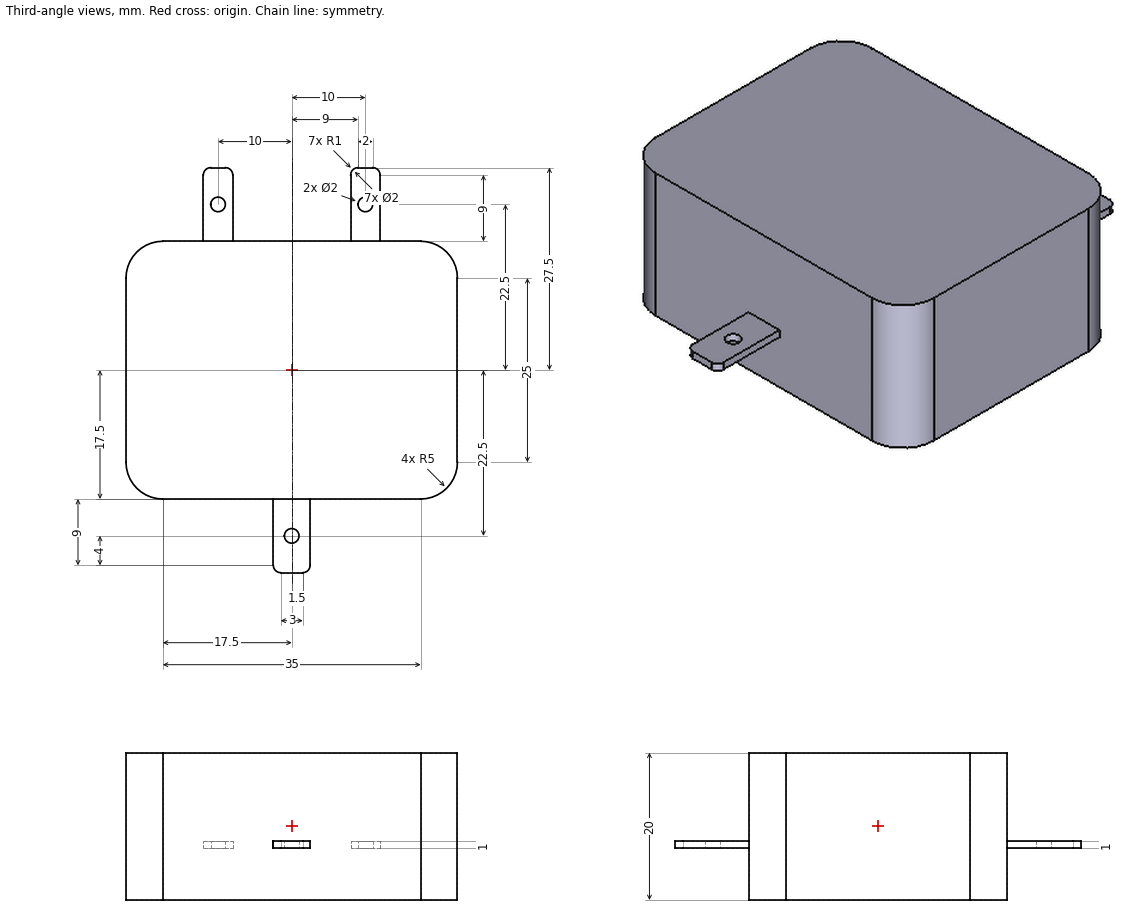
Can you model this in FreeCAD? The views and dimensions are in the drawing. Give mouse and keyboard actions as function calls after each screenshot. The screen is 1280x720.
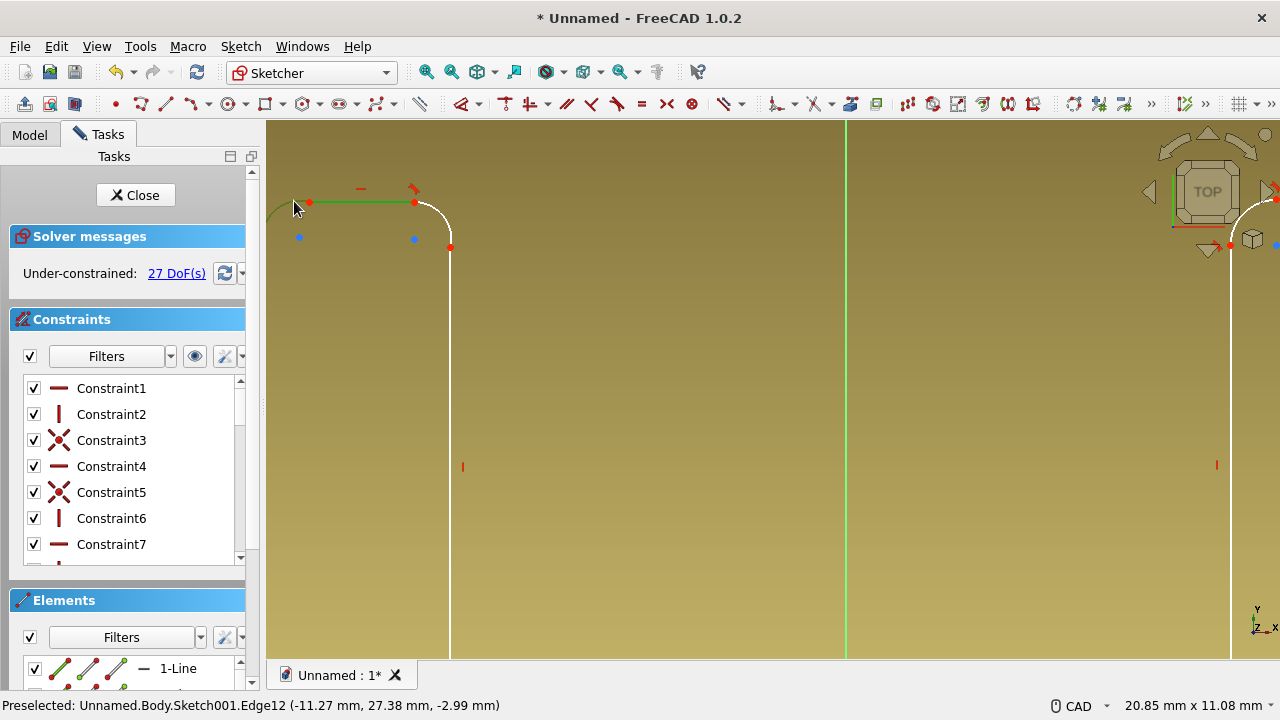
click(617, 104)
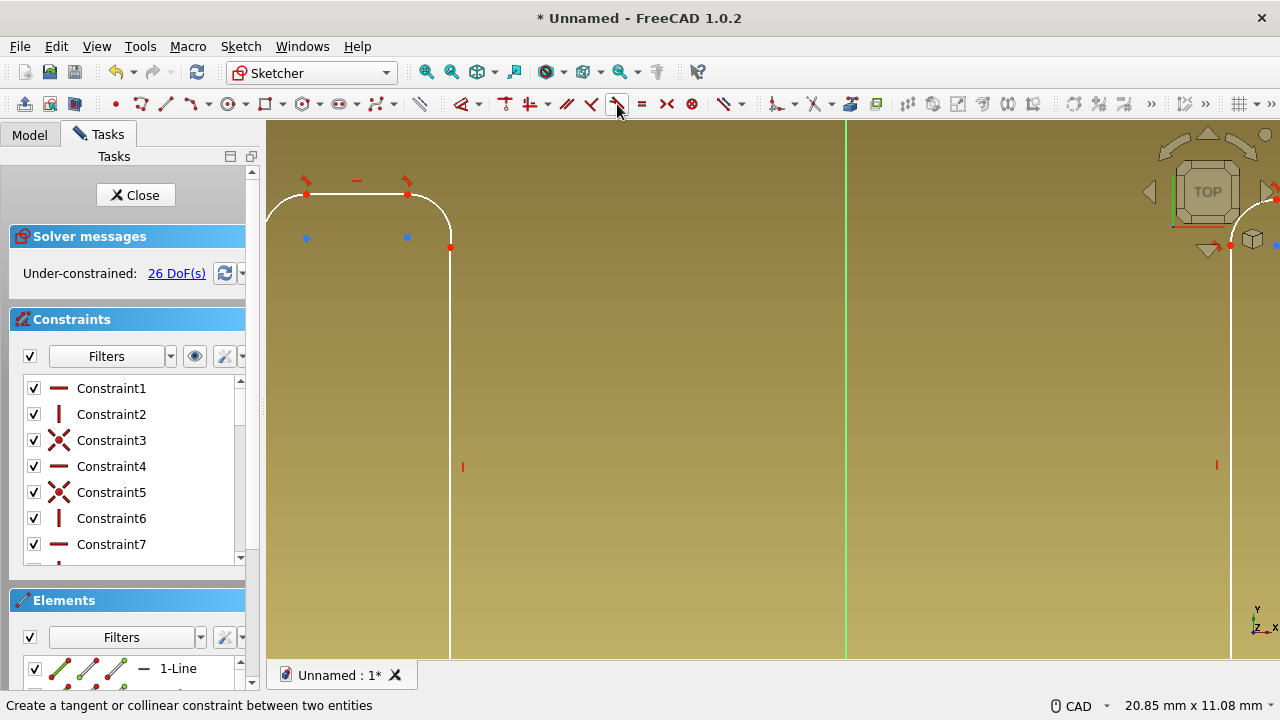
scroll(682, 211, down, 10)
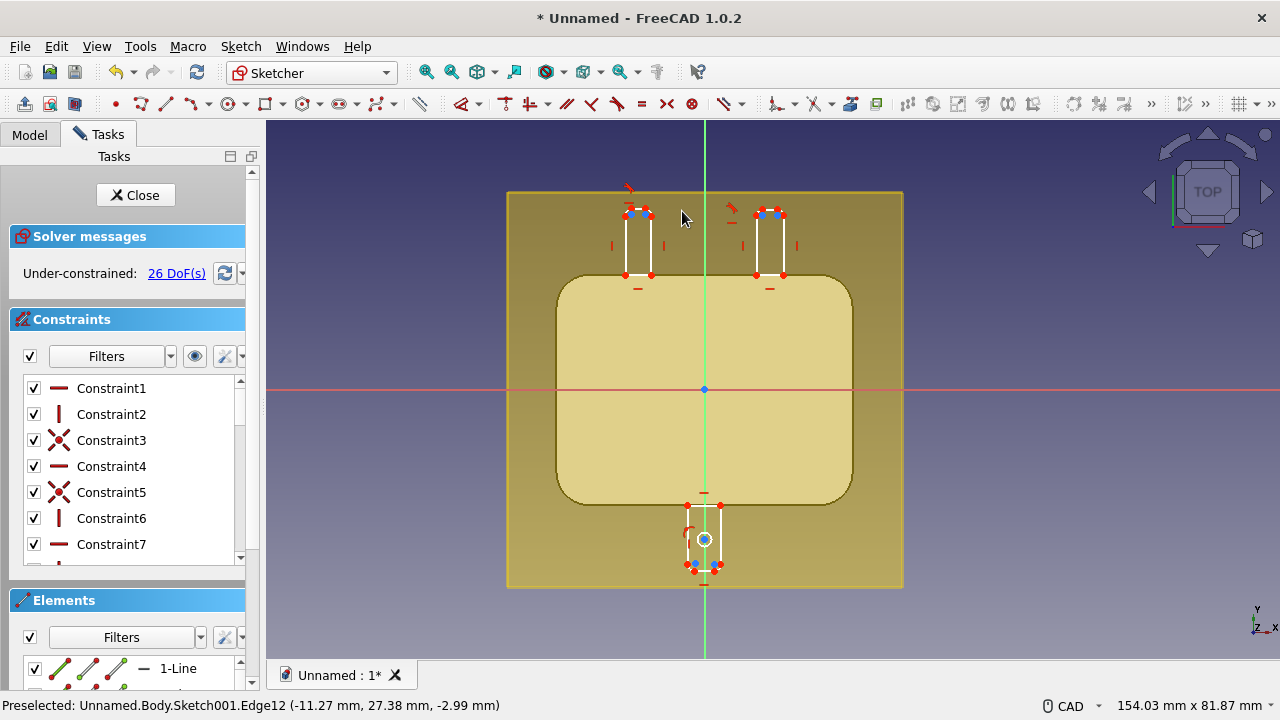
click(651, 234)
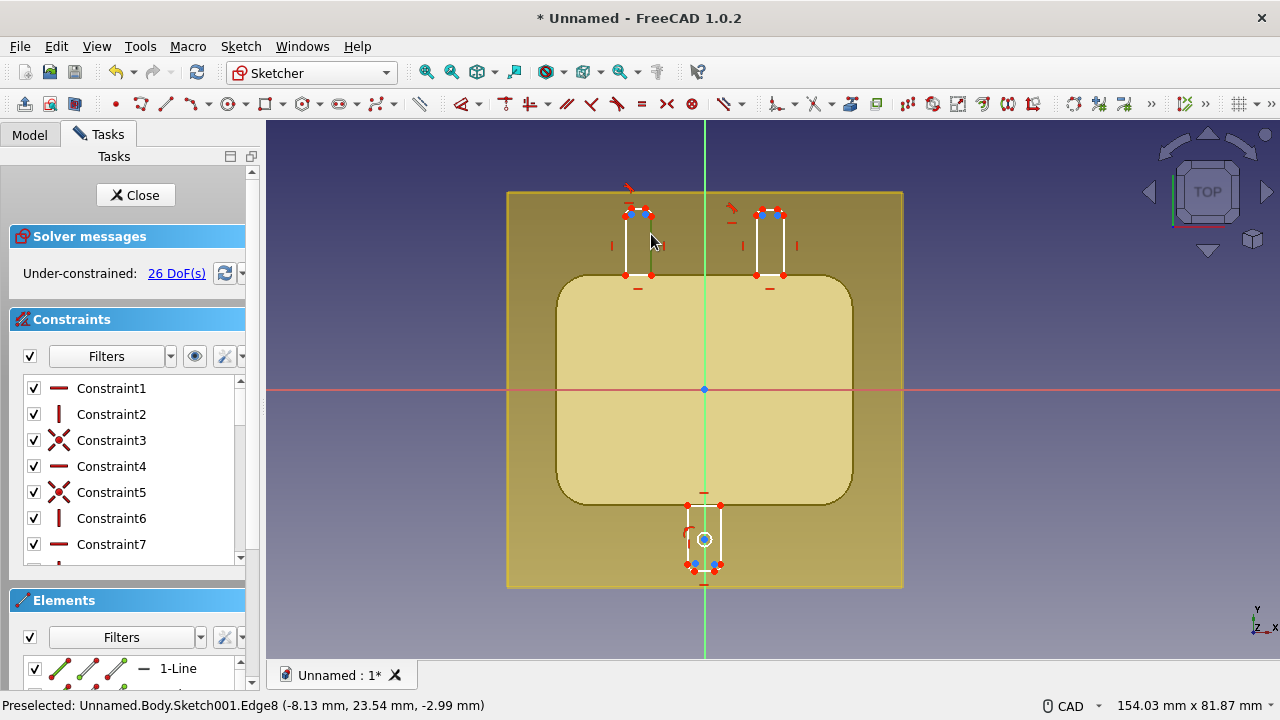
scroll(650, 211, up, 5)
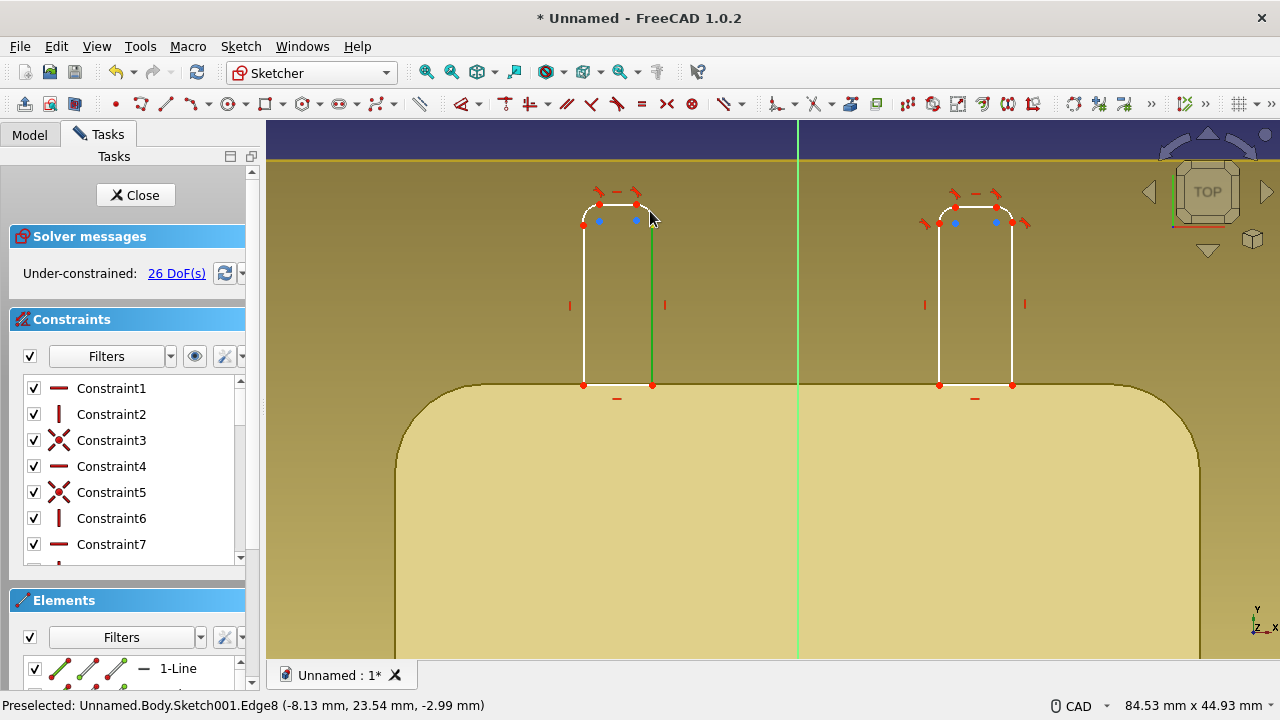
click(649, 211)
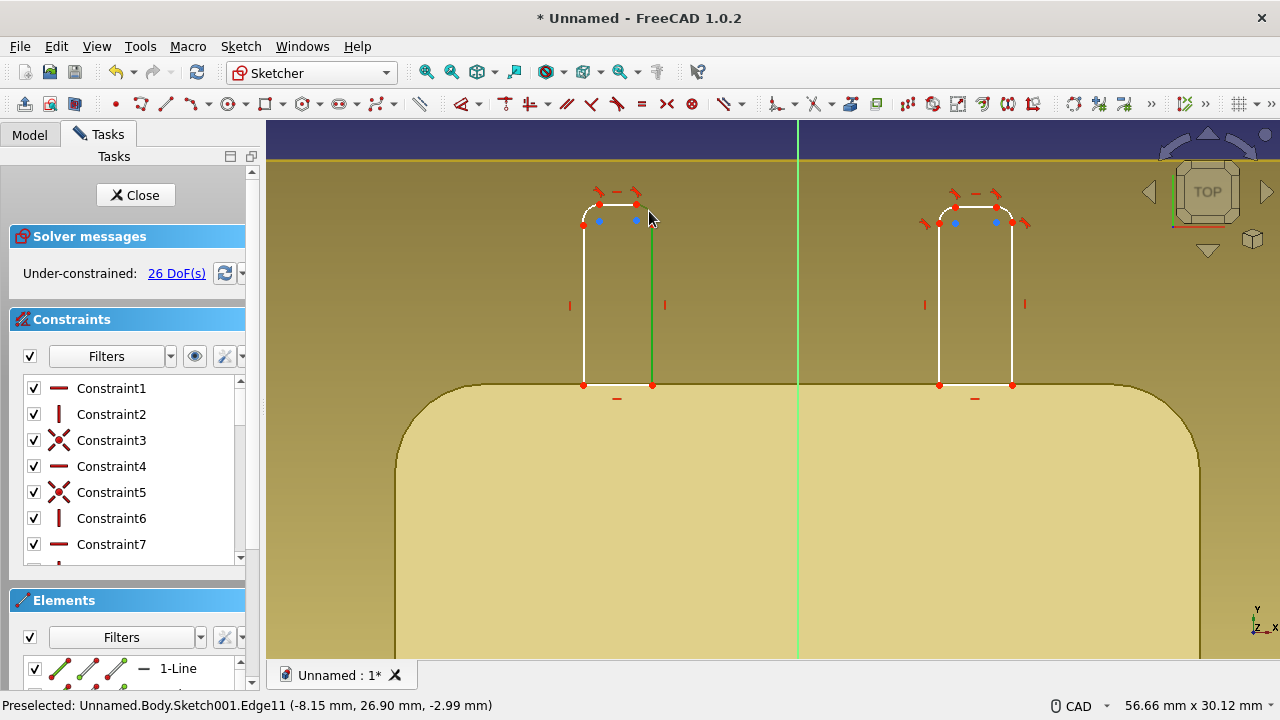
click(617, 104)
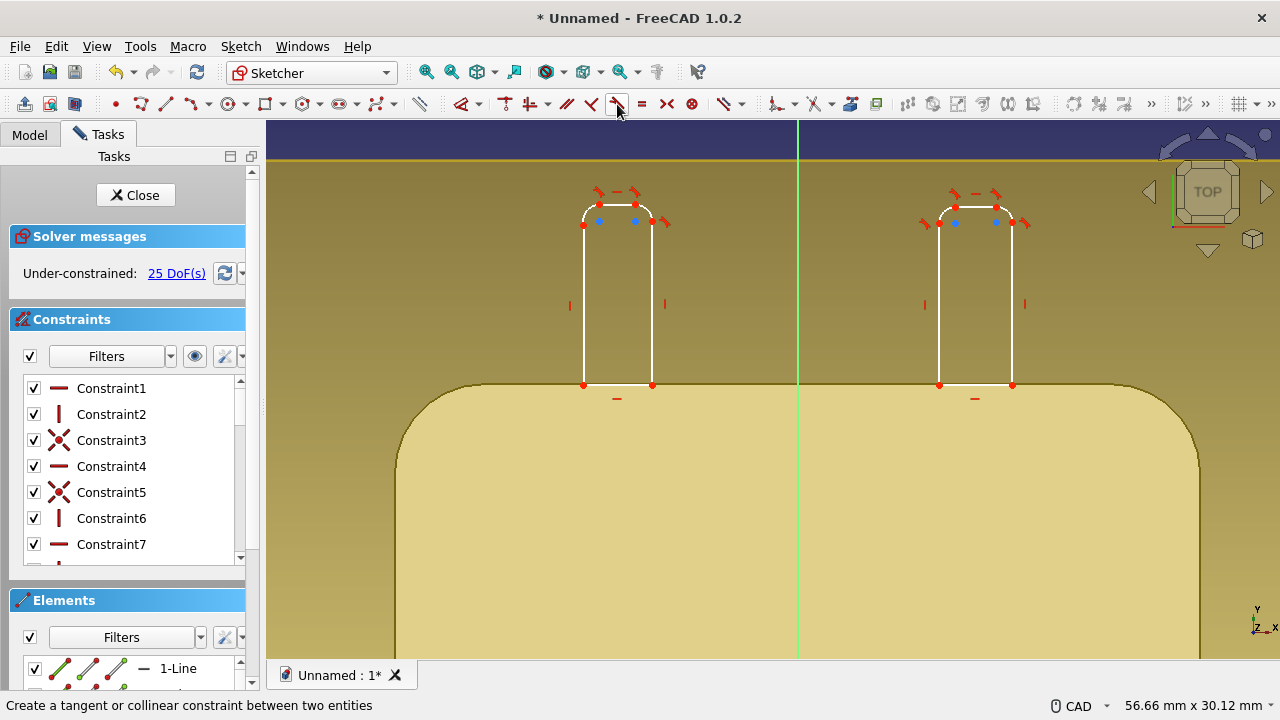
click(584, 337)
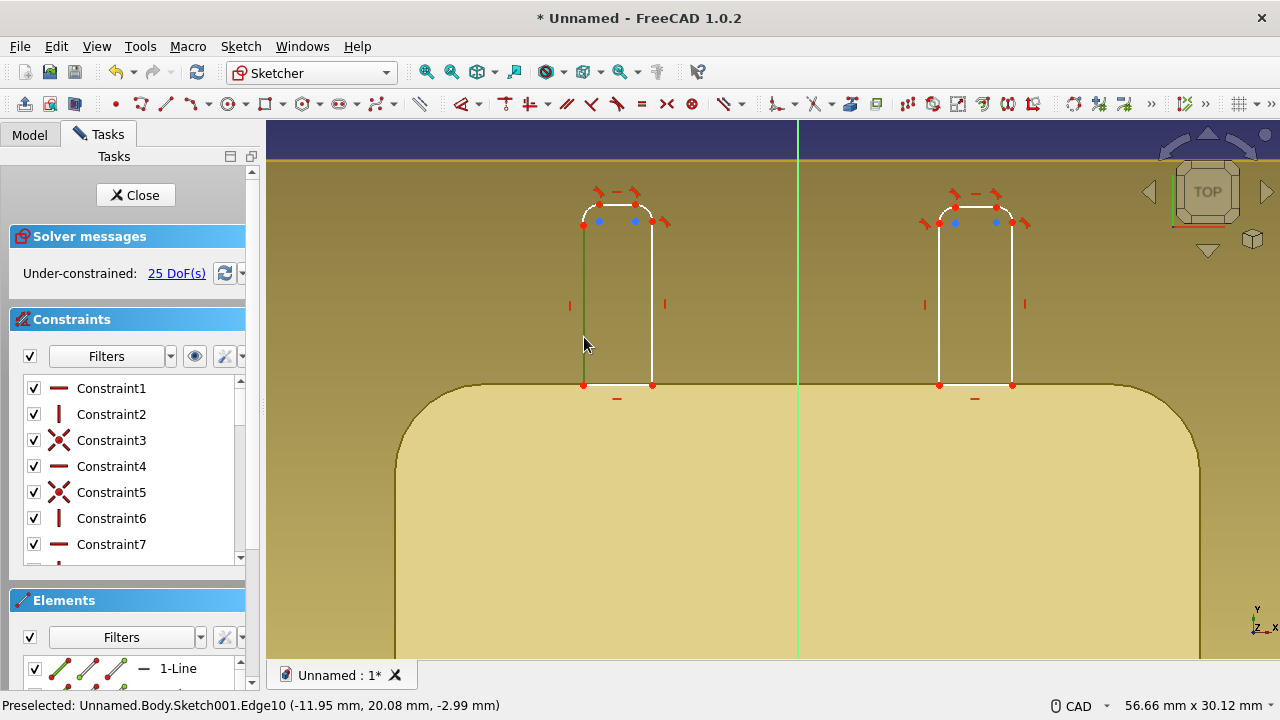
click(587, 211)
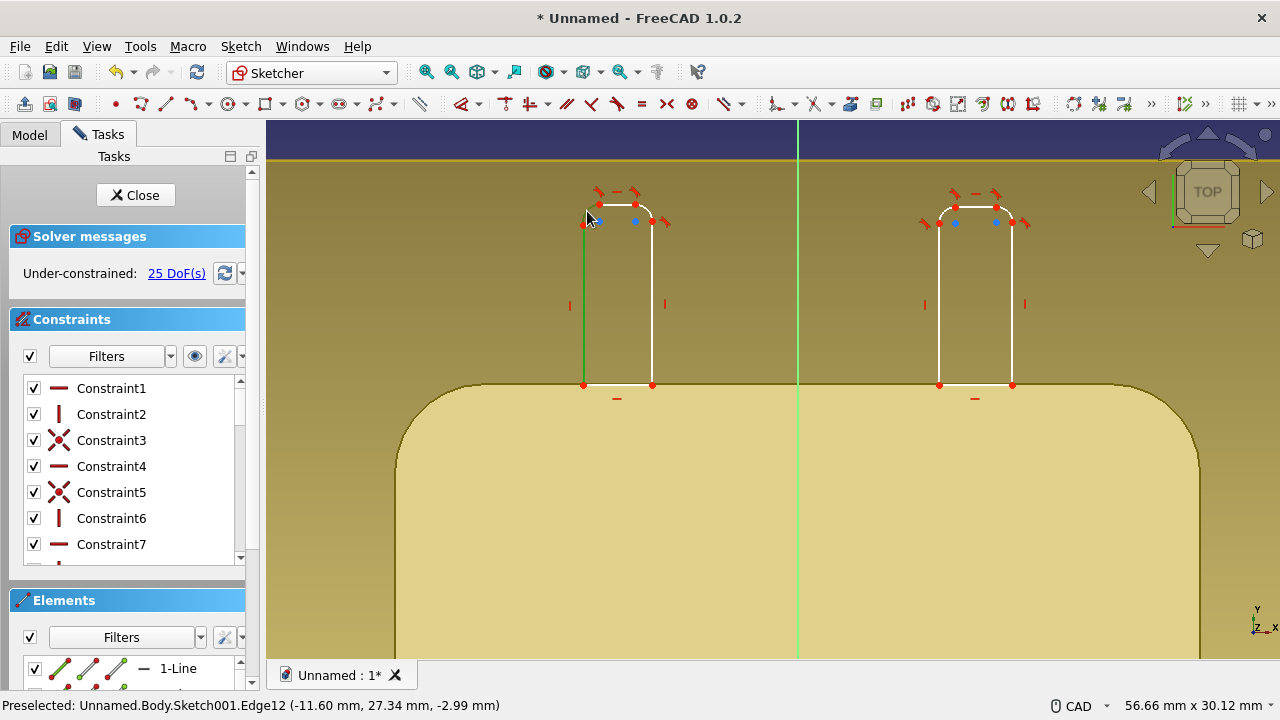
key(t)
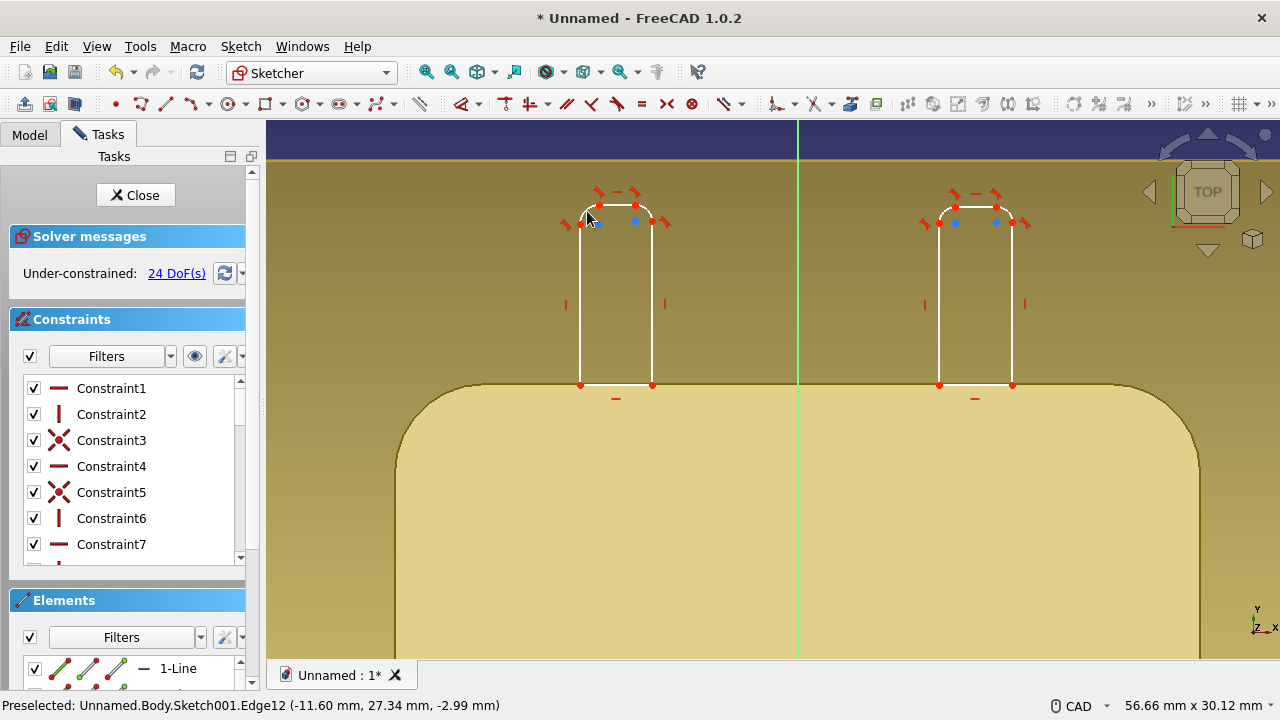
scroll(650, 210, down, 5)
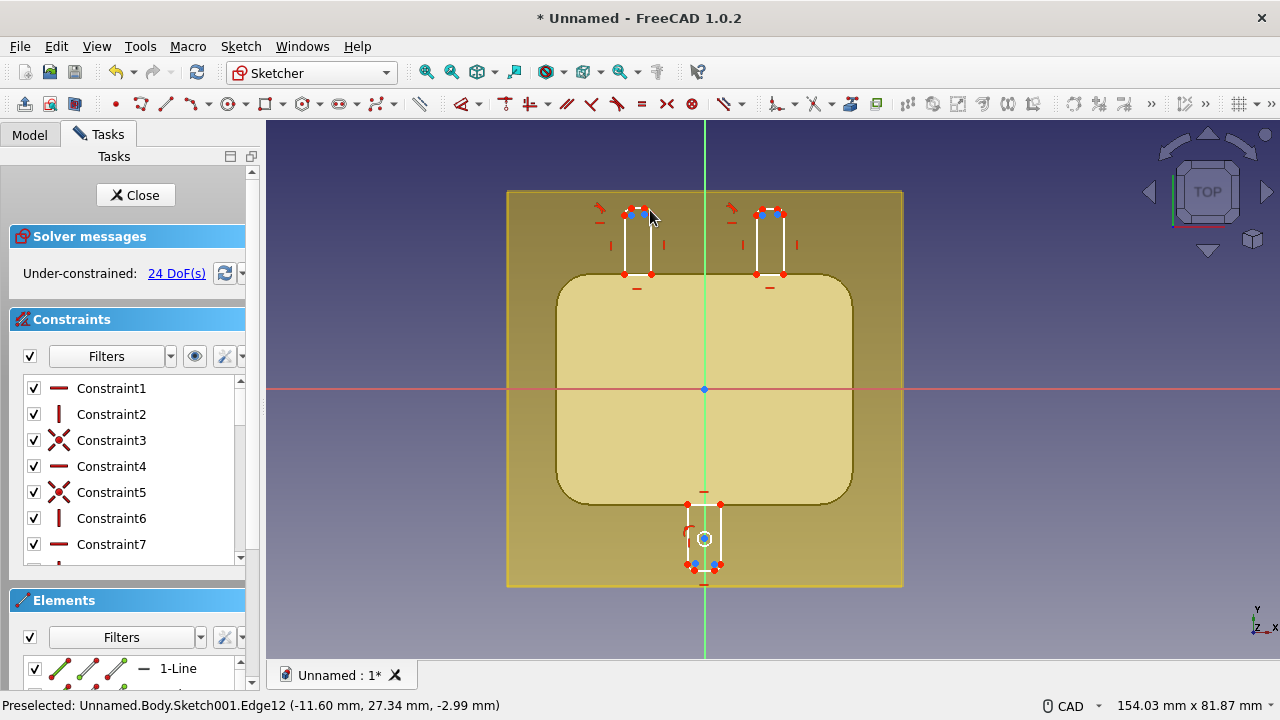
scroll(708, 571, up, 7)